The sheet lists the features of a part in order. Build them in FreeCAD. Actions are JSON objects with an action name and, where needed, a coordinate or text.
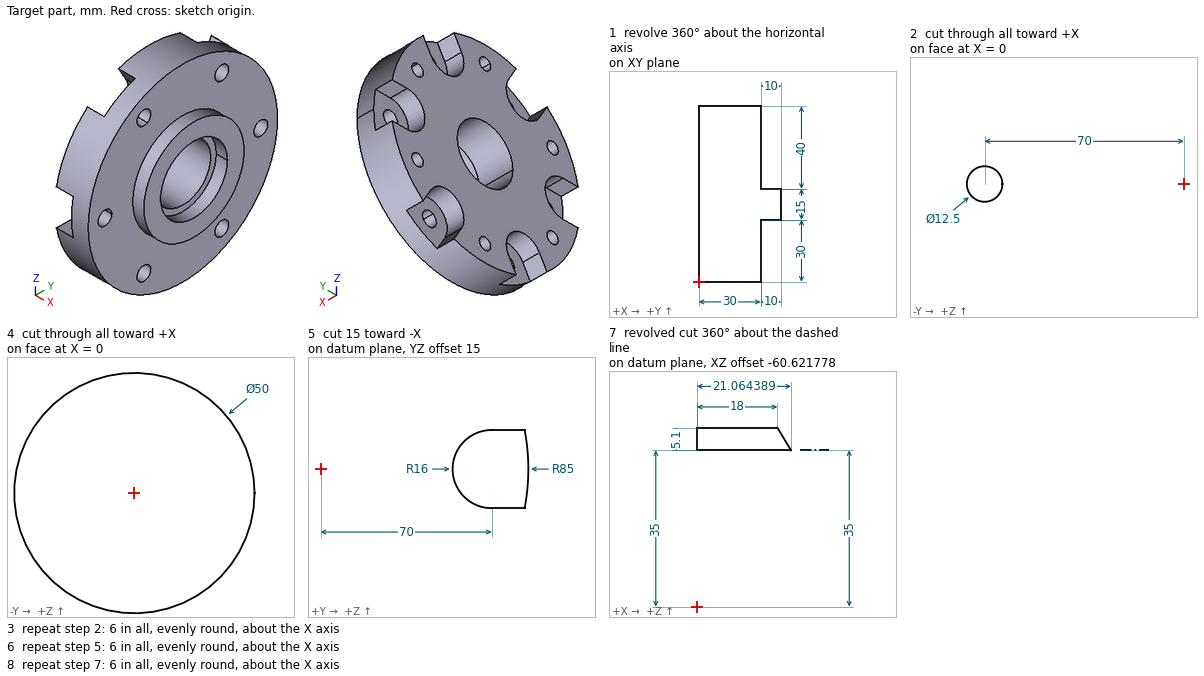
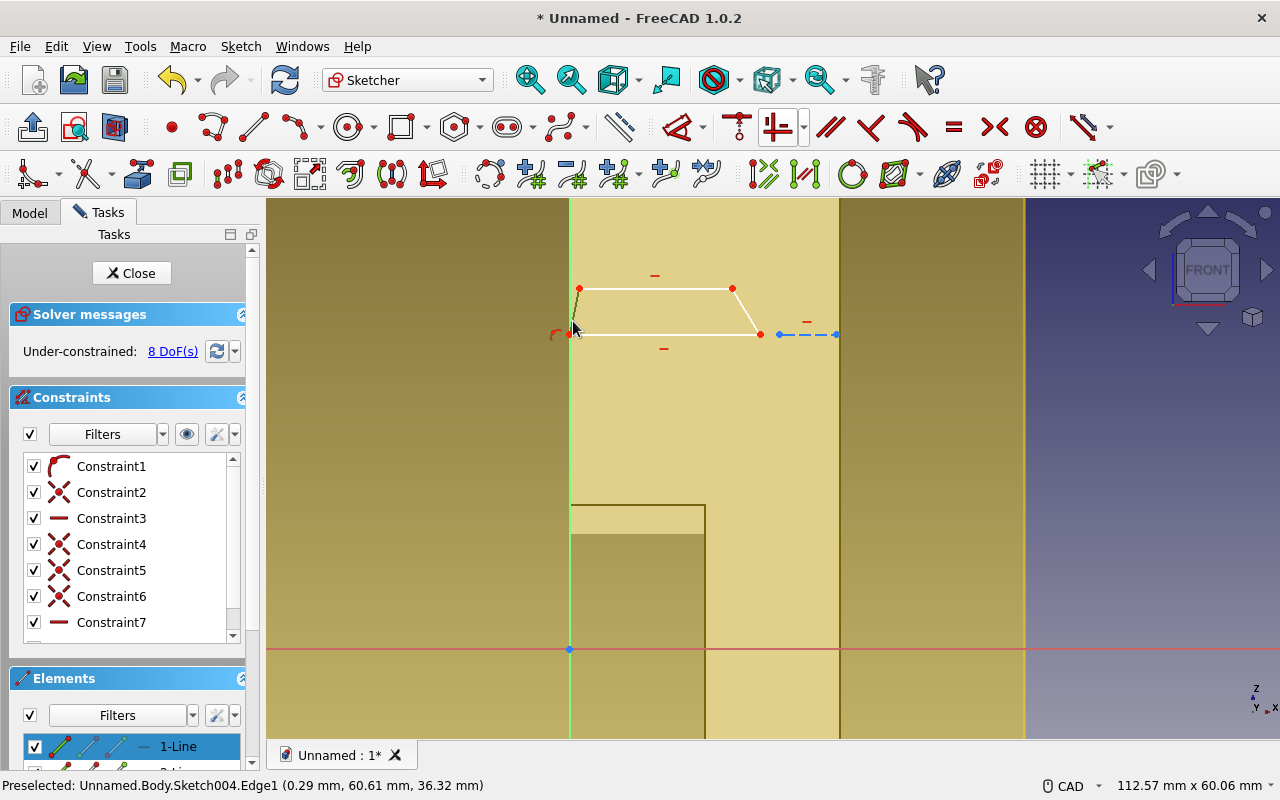
{"action": "key", "text": "v"}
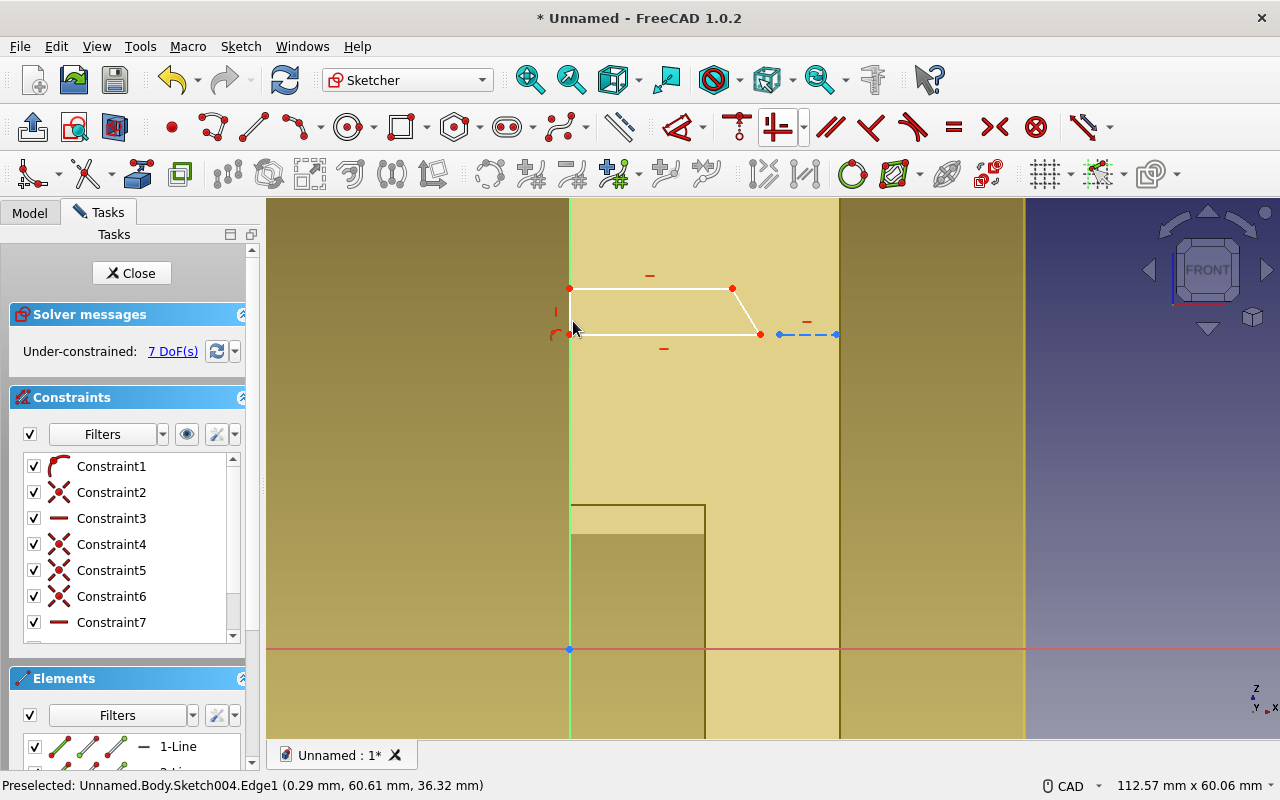
{"action": "left_click", "coordinate": [676, 128]}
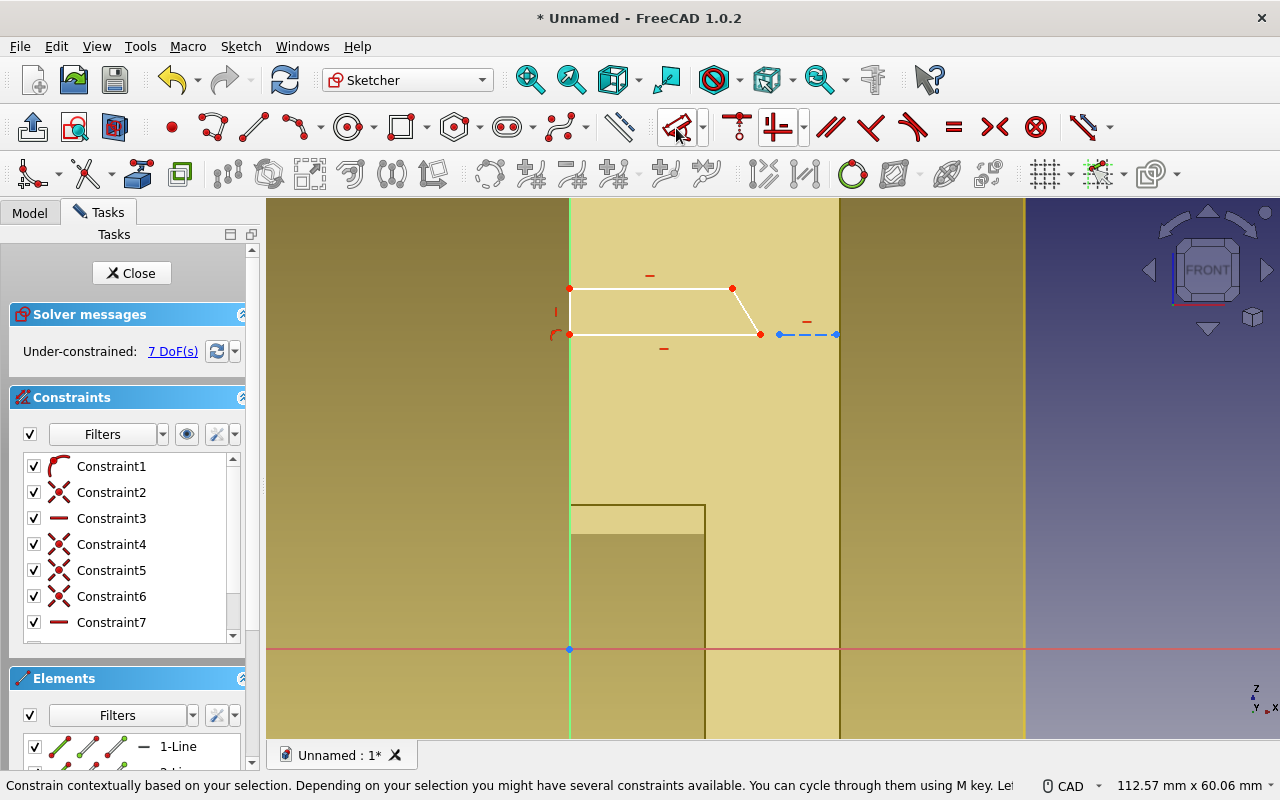
{"action": "left_click", "coordinate": [619, 289]}
{"action": "left_click", "coordinate": [651, 255]}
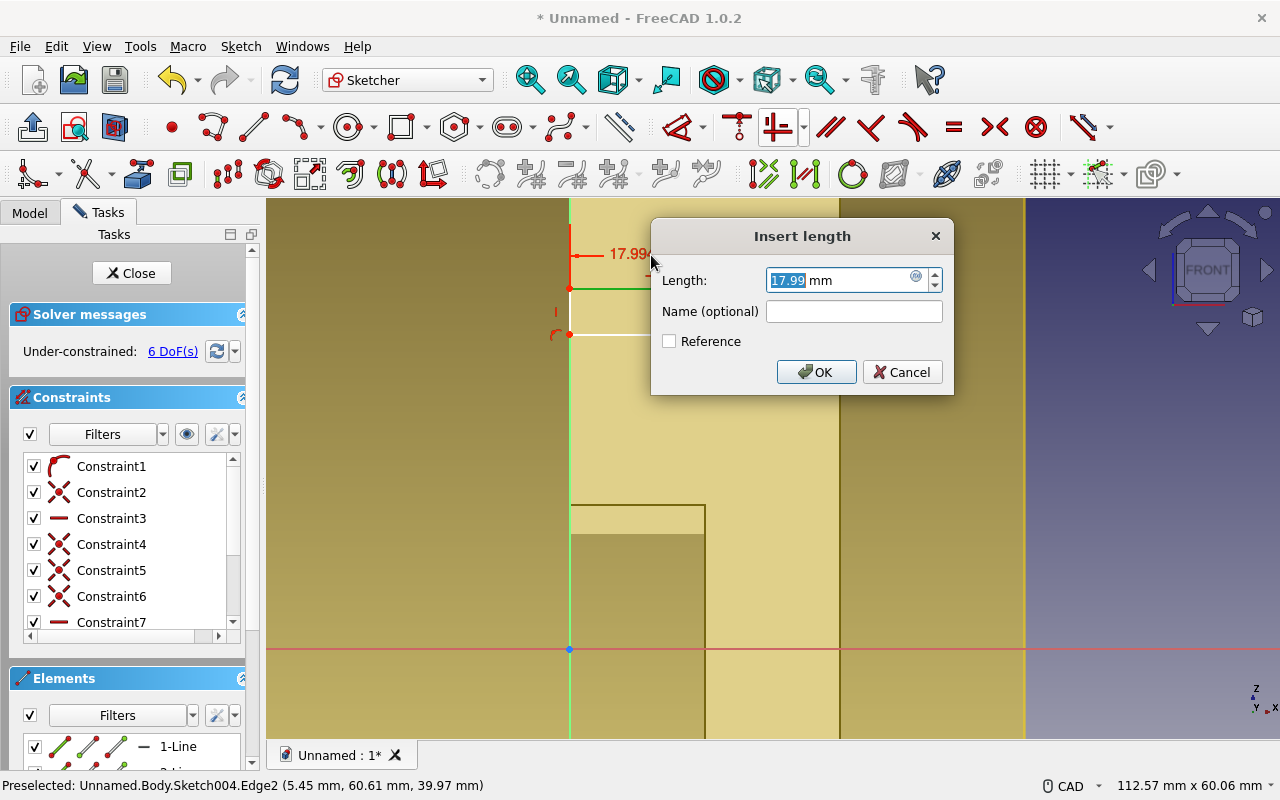
{"action": "type", "text": "18"}
{"action": "key", "text": "Return"}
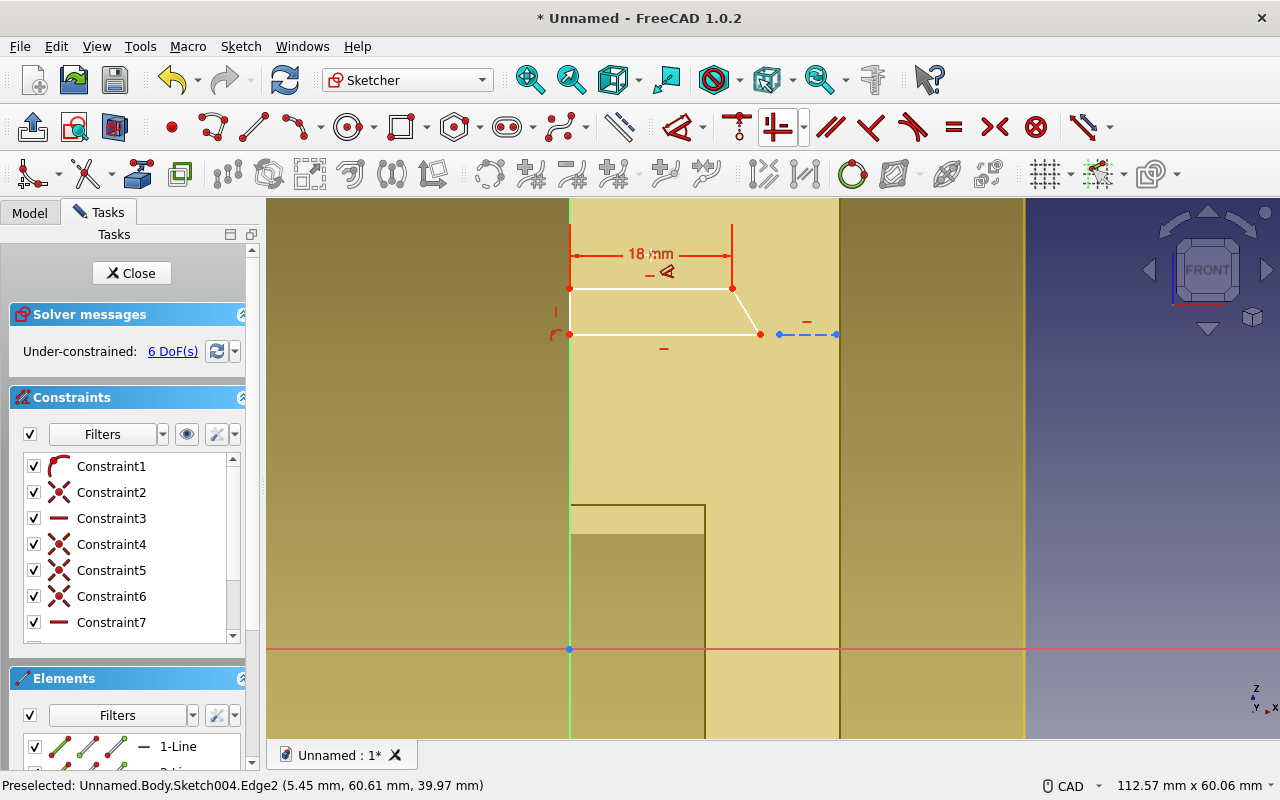
{"action": "left_click", "coordinate": [570, 321]}
{"action": "left_click", "coordinate": [536, 312]}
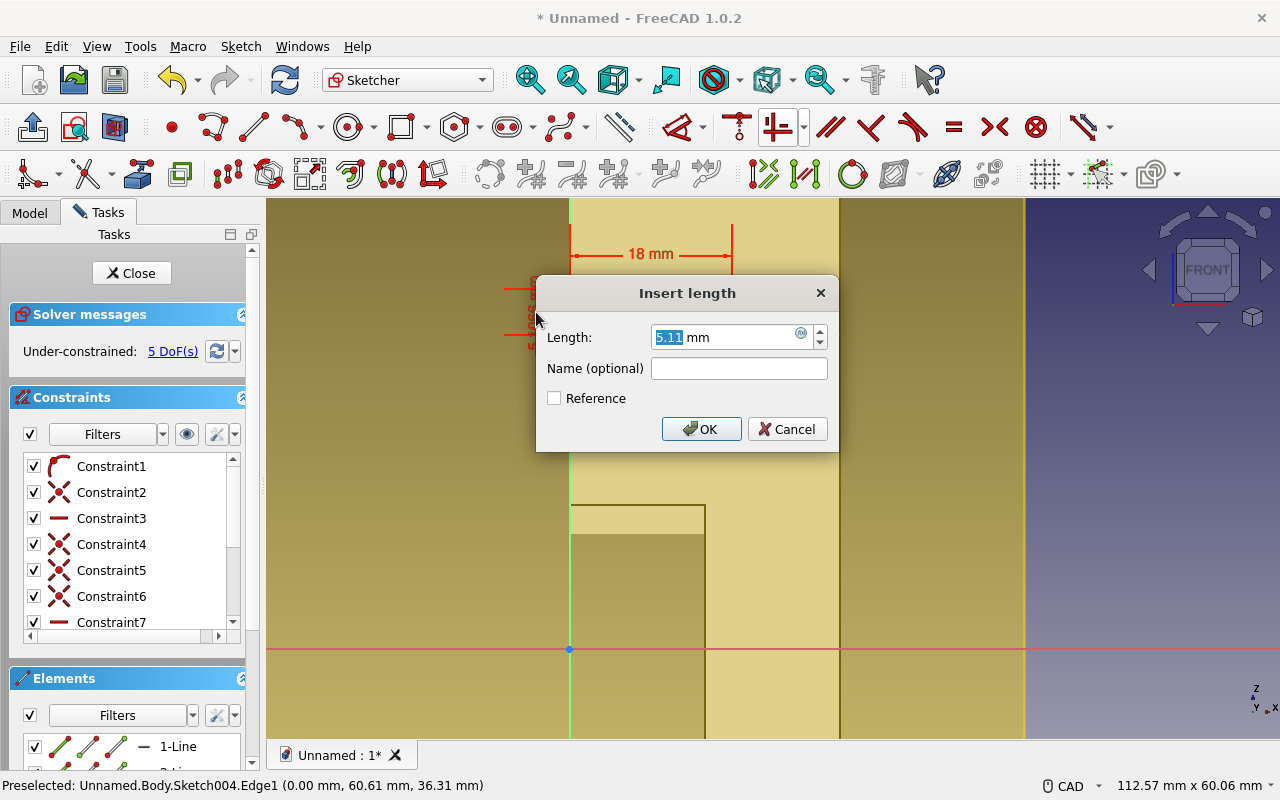
{"action": "type", "text": "5.1"}
{"action": "key", "text": "Return"}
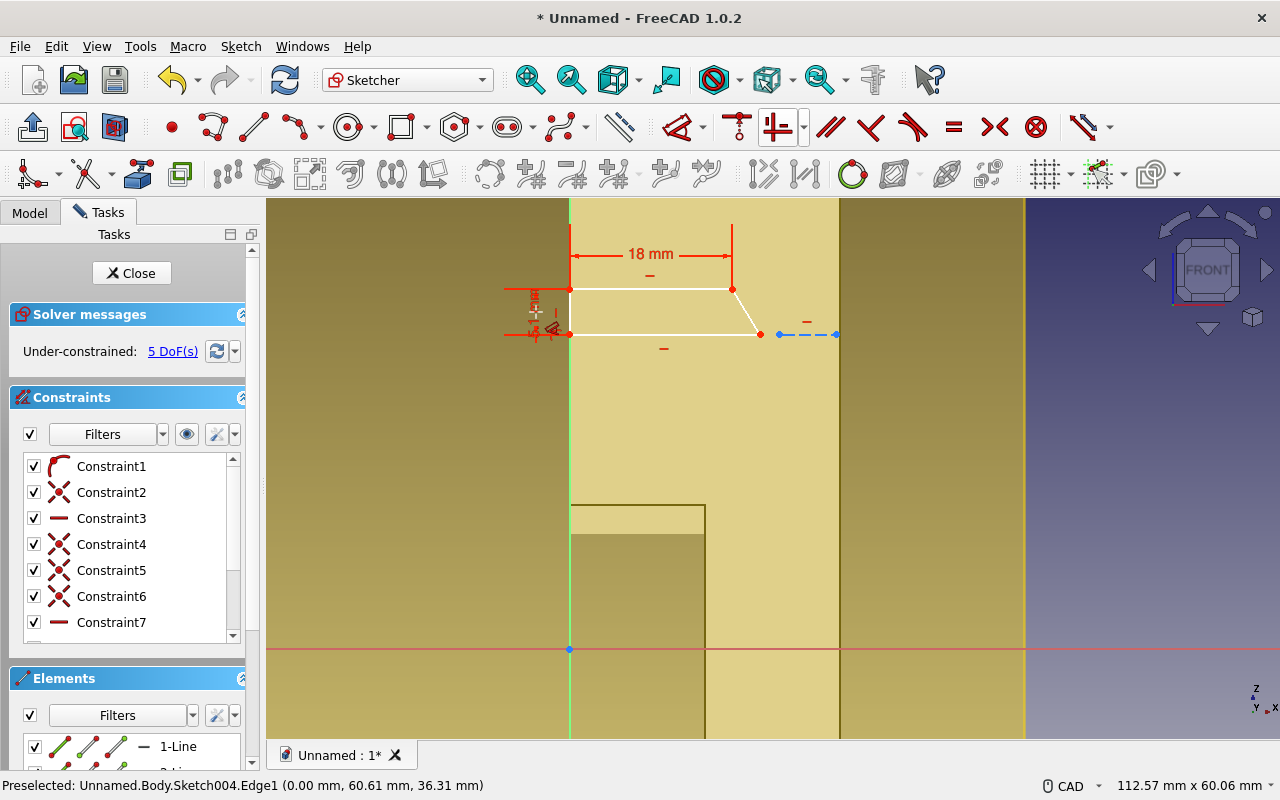
{"action": "left_click", "coordinate": [570, 335]}
{"action": "left_click", "coordinate": [536, 492]}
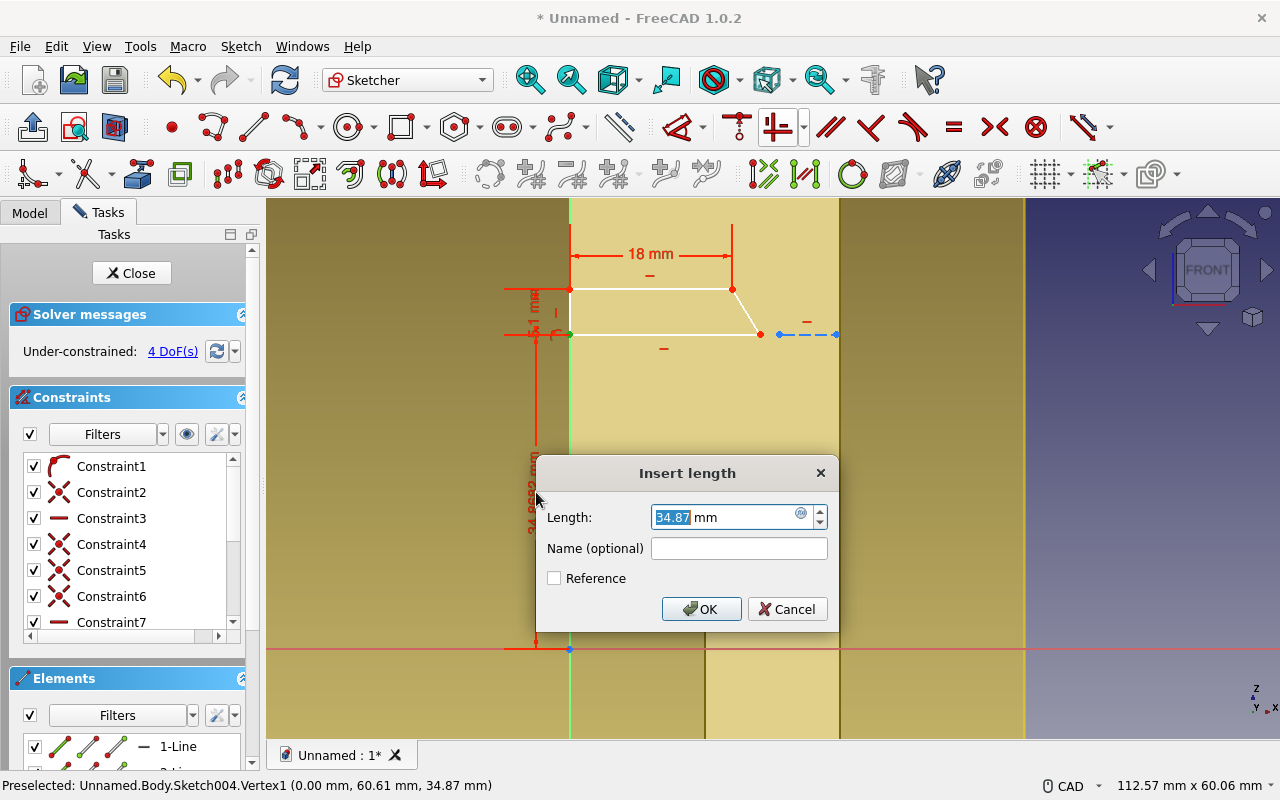
{"action": "type", "text": "35"}
{"action": "key", "text": "Return"}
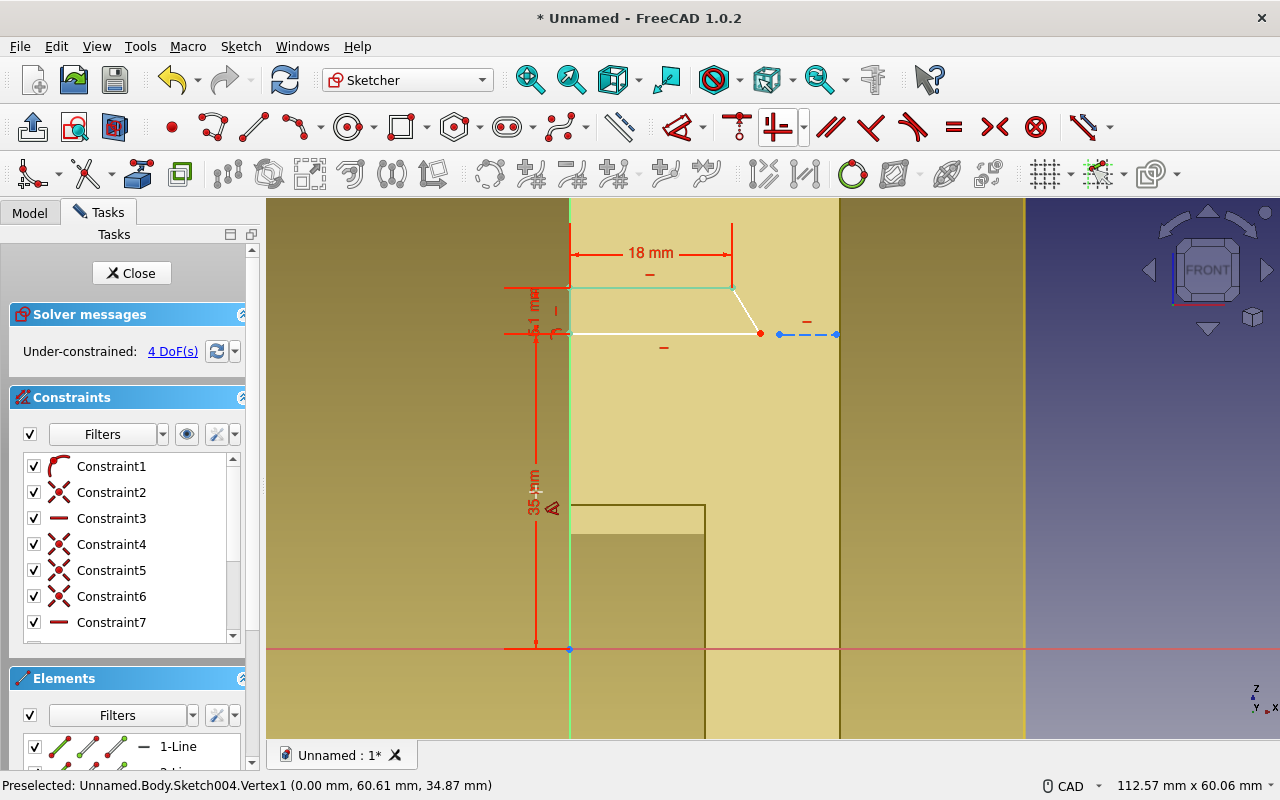
{"action": "left_click", "coordinate": [779, 335]}
{"action": "left_click", "coordinate": [536, 420]}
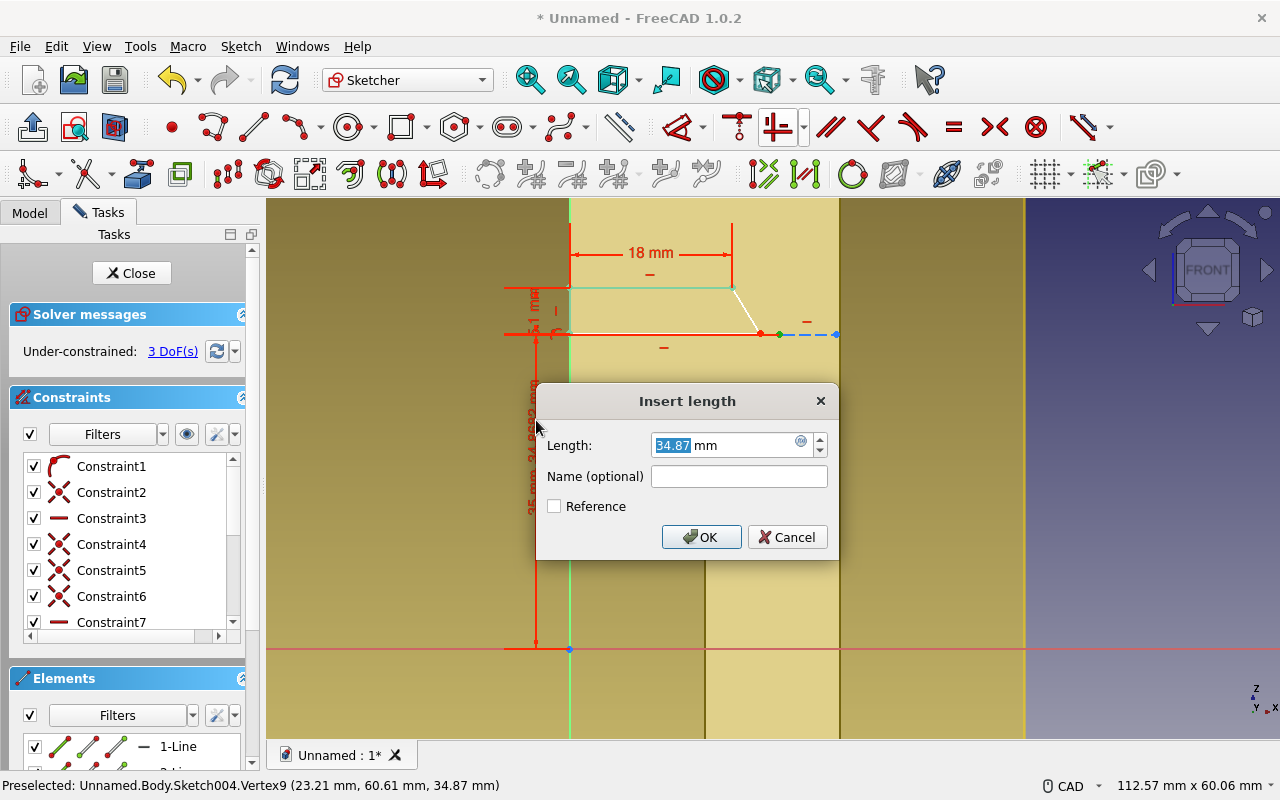
{"action": "type", "text": "35"}
{"action": "key", "text": "Return"}